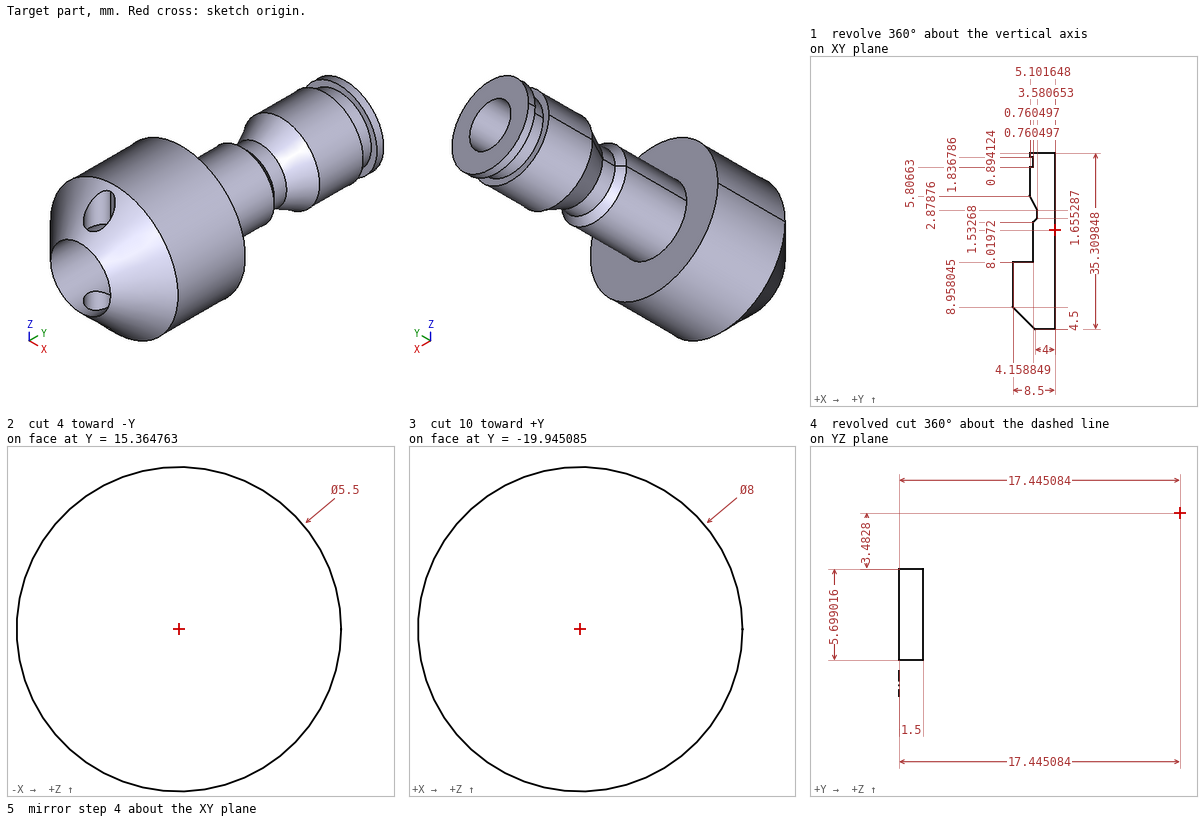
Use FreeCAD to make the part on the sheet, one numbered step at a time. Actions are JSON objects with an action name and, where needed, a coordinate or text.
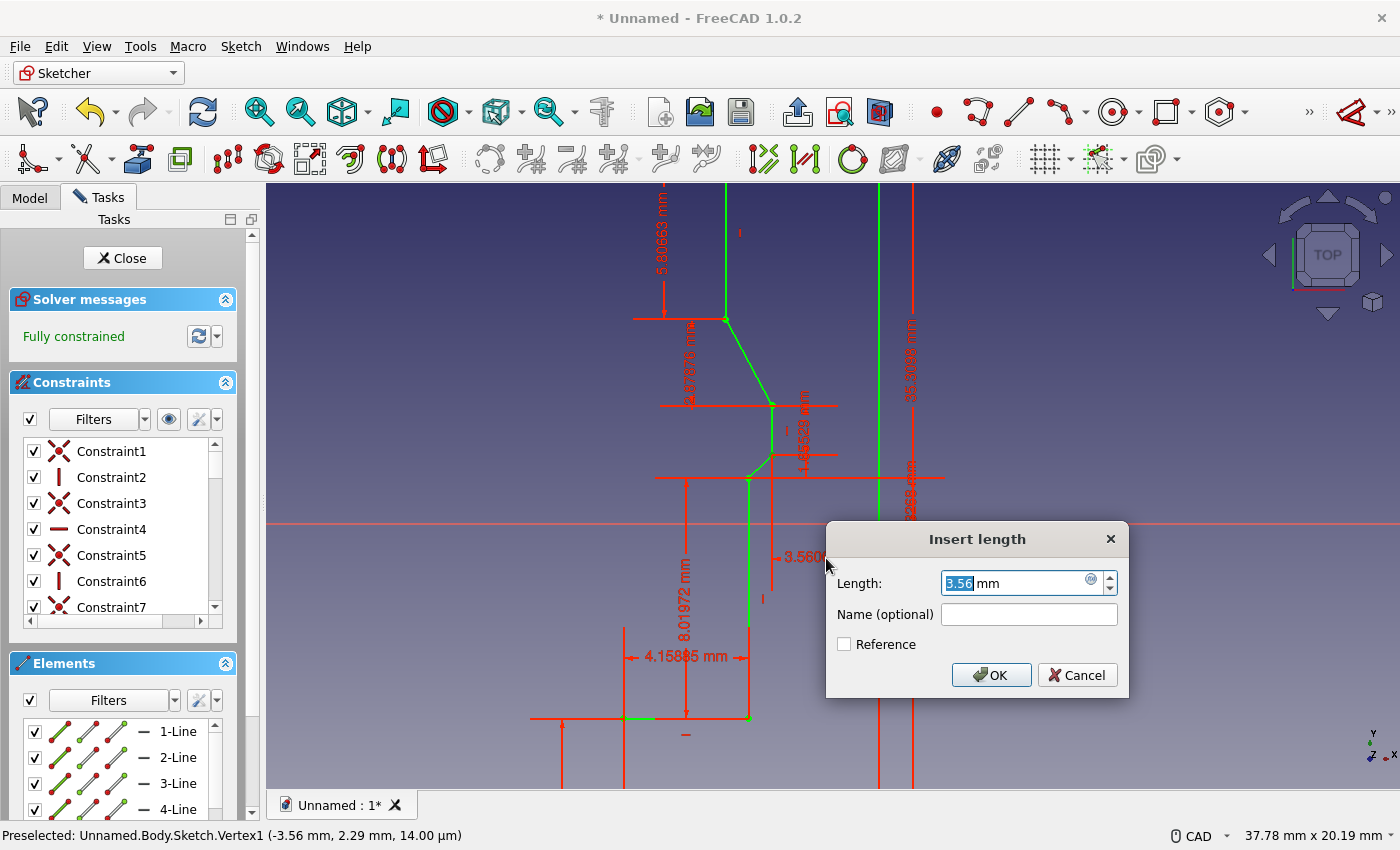
{"action": "type", "text": "3.580653"}
{"action": "key", "text": "Return"}
{"action": "key", "text": "Escape"}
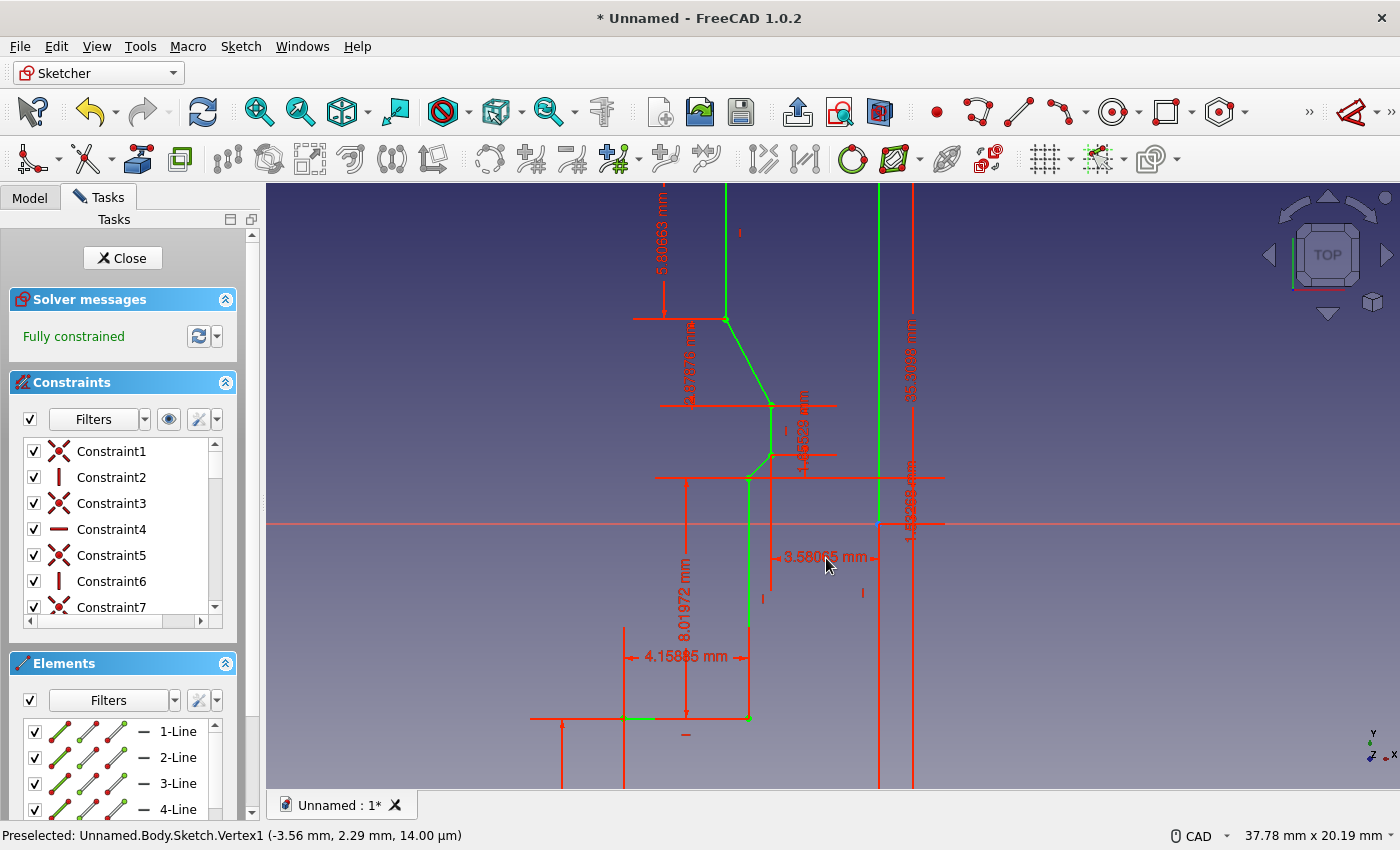
{"action": "left_click", "coordinate": [123, 258]}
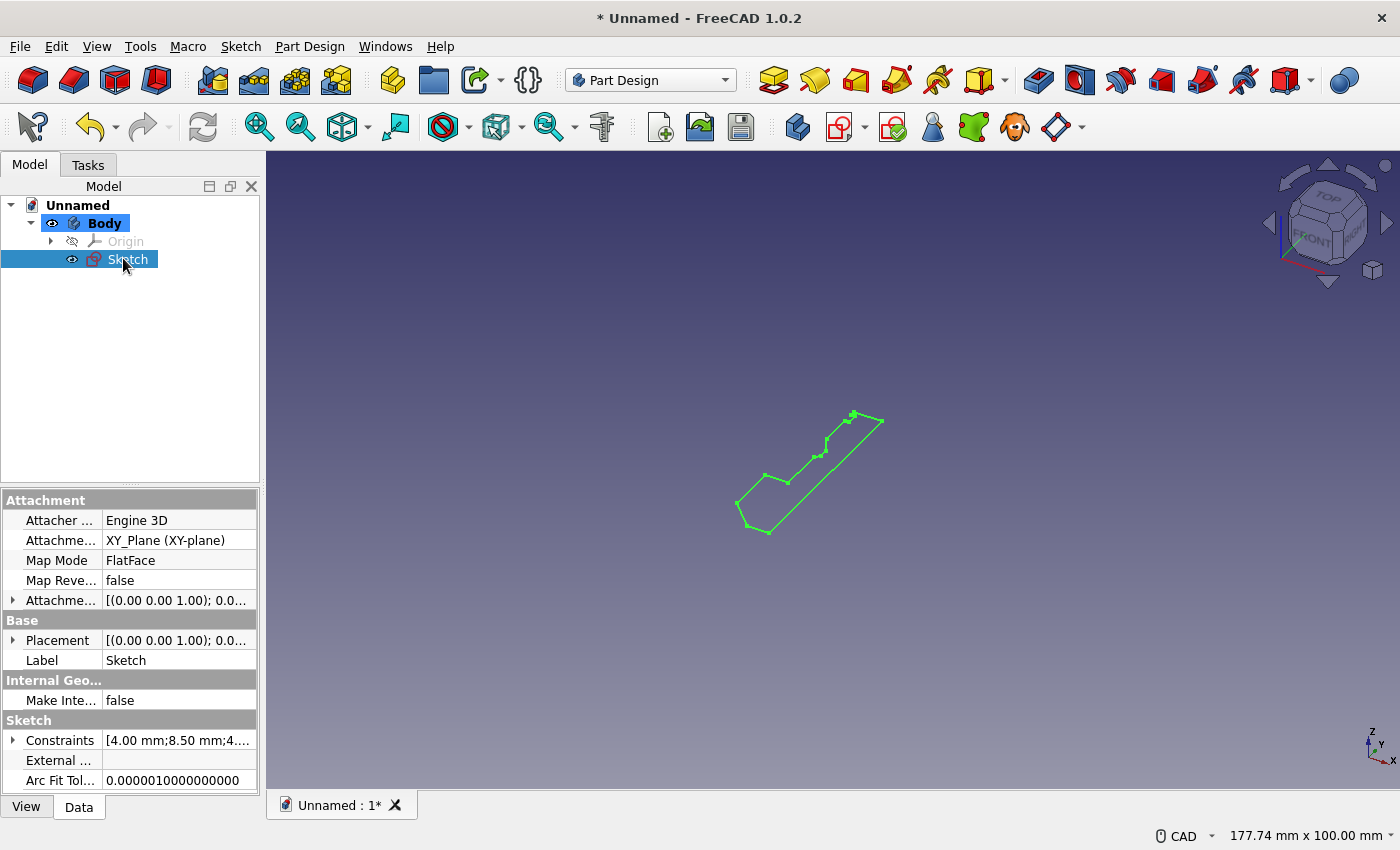
{"action": "left_click", "coordinate": [815, 80]}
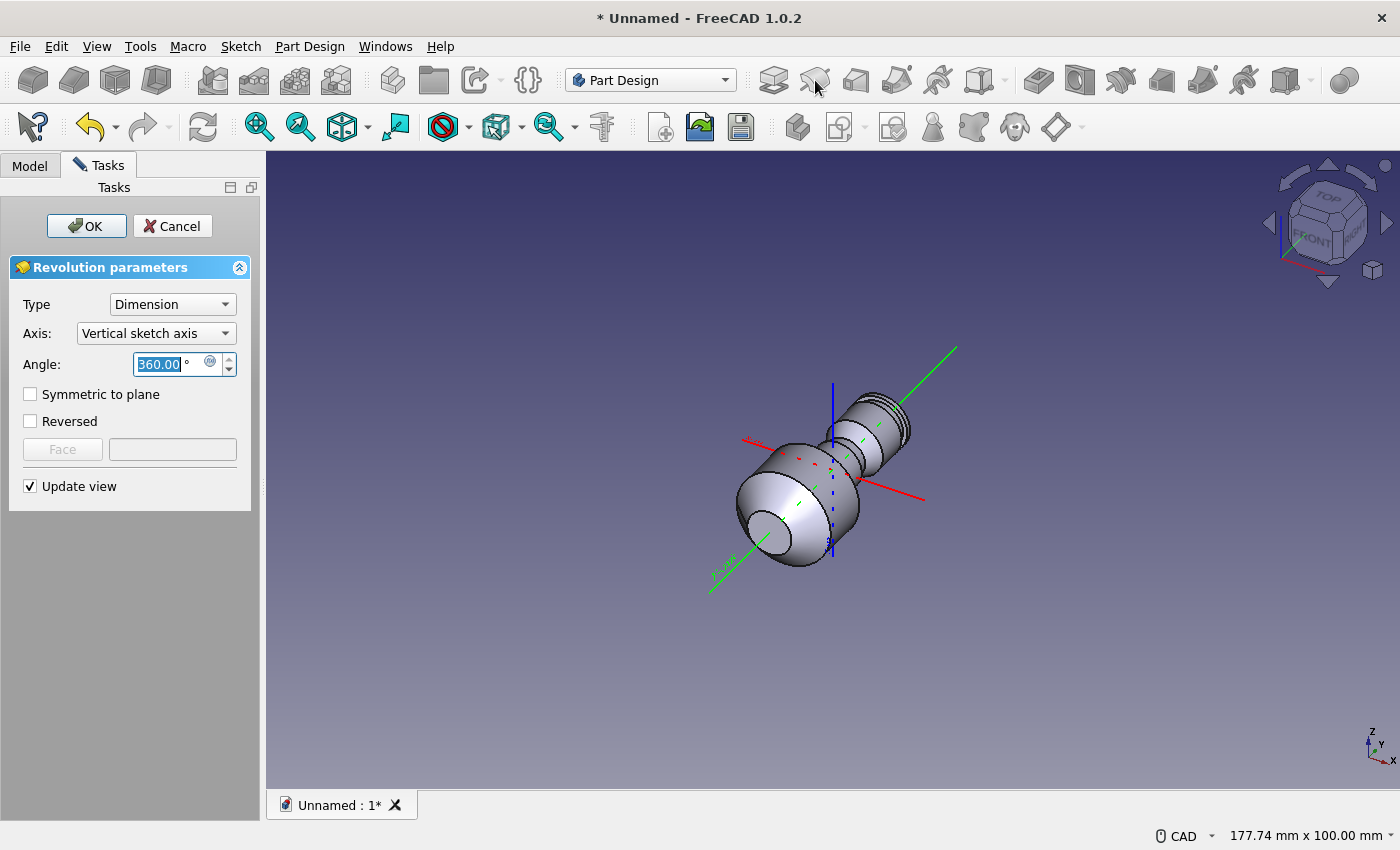
{"action": "left_click", "coordinate": [87, 226]}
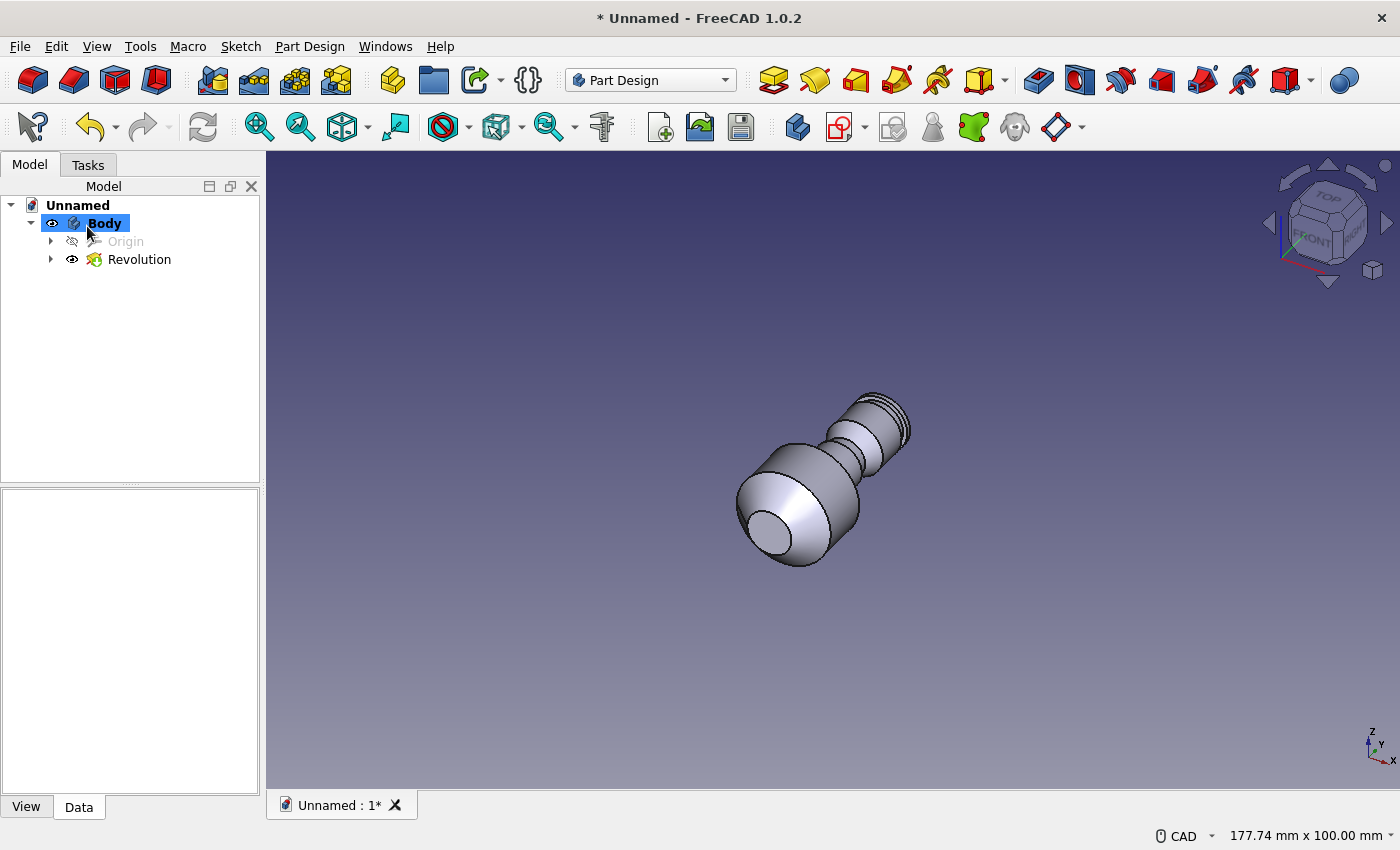
{"action": "left_click", "coordinate": [260, 128]}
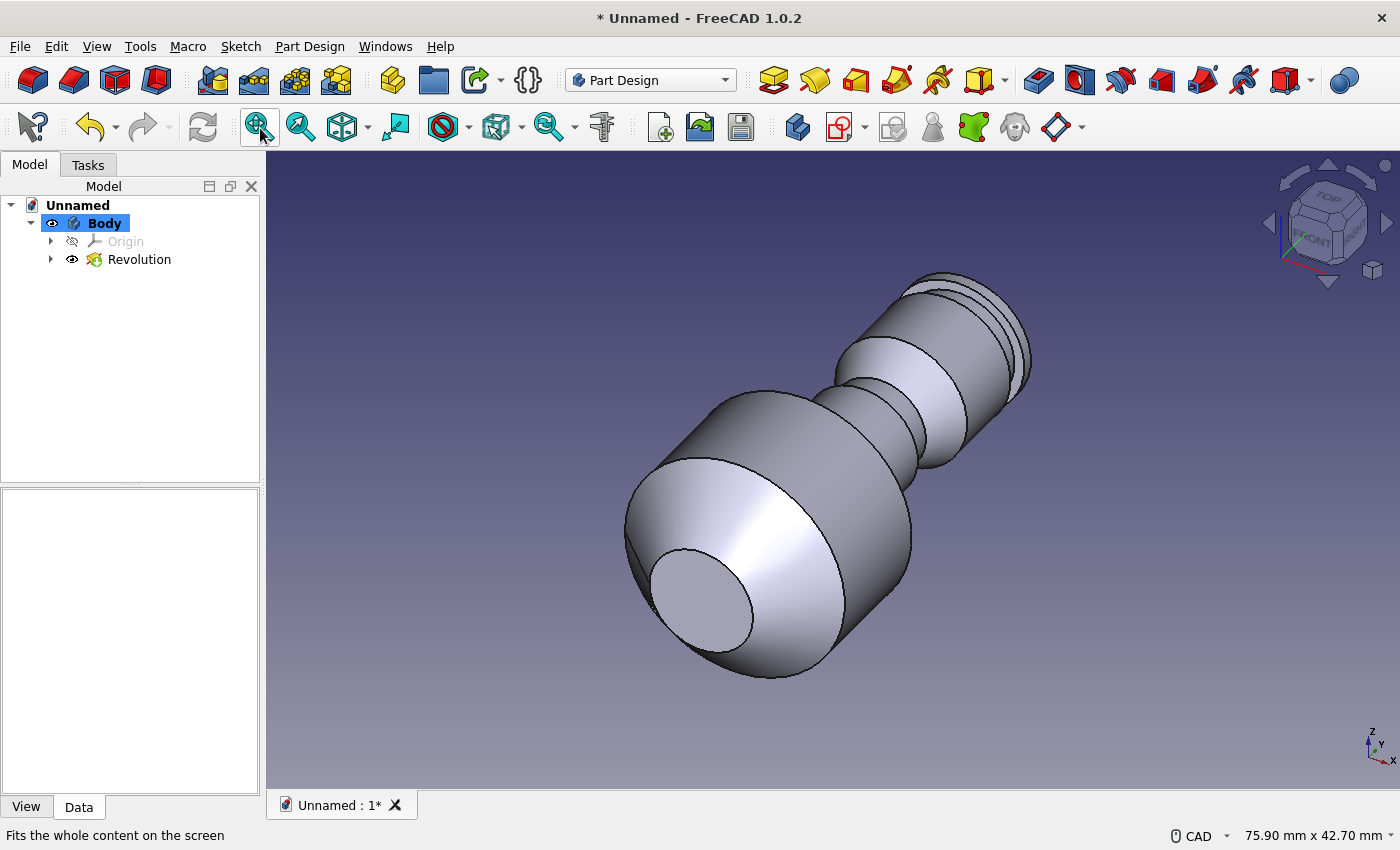
{"action": "key", "text": "4"}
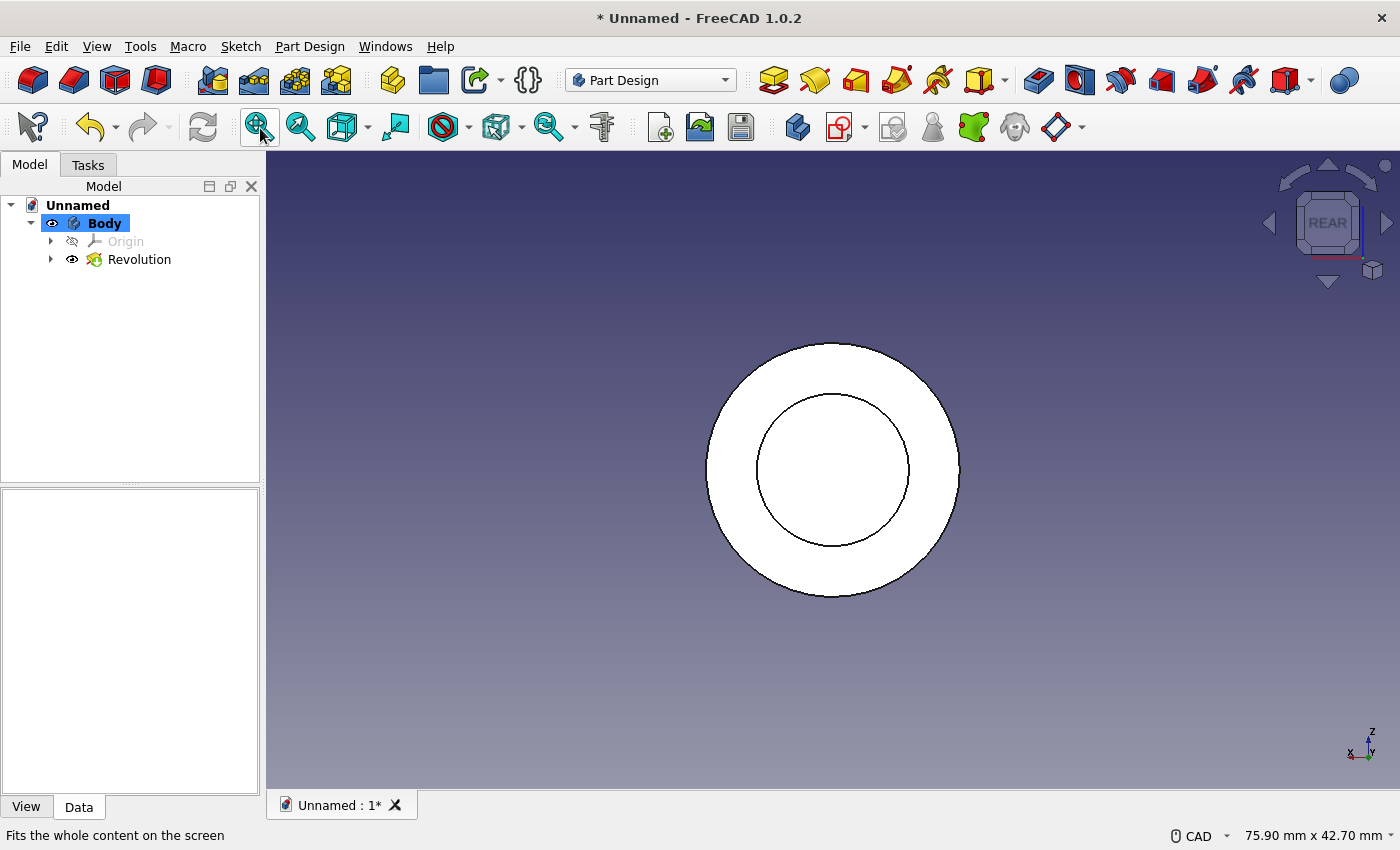
{"action": "left_click", "coordinate": [260, 128]}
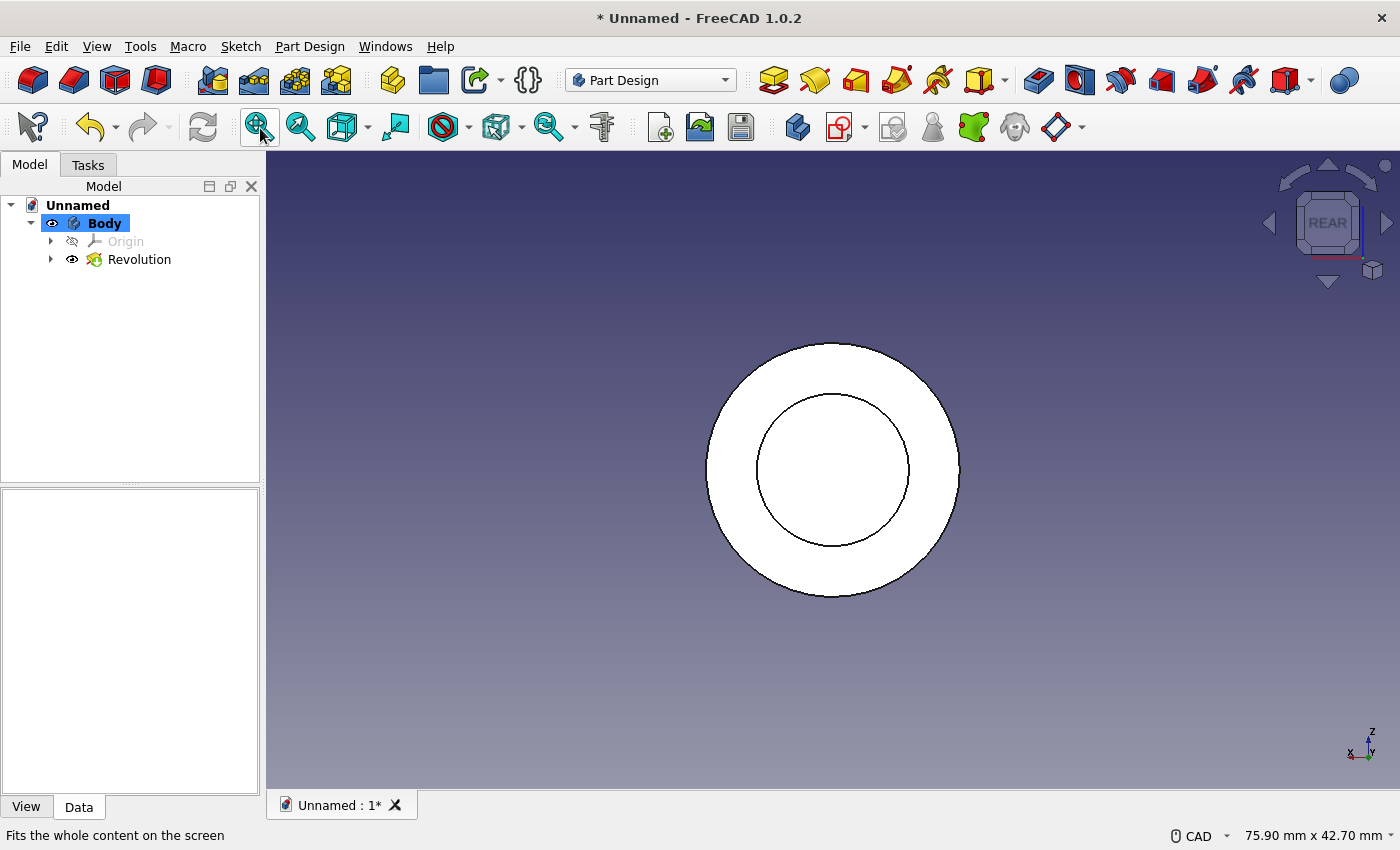
{"action": "left_click", "coordinate": [833, 469]}